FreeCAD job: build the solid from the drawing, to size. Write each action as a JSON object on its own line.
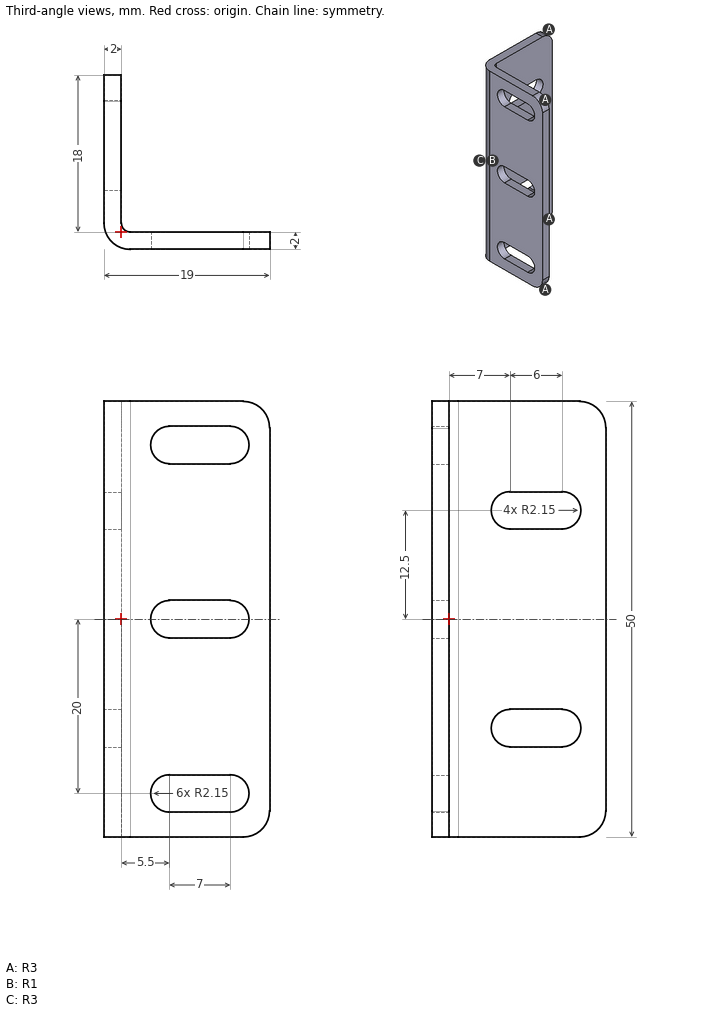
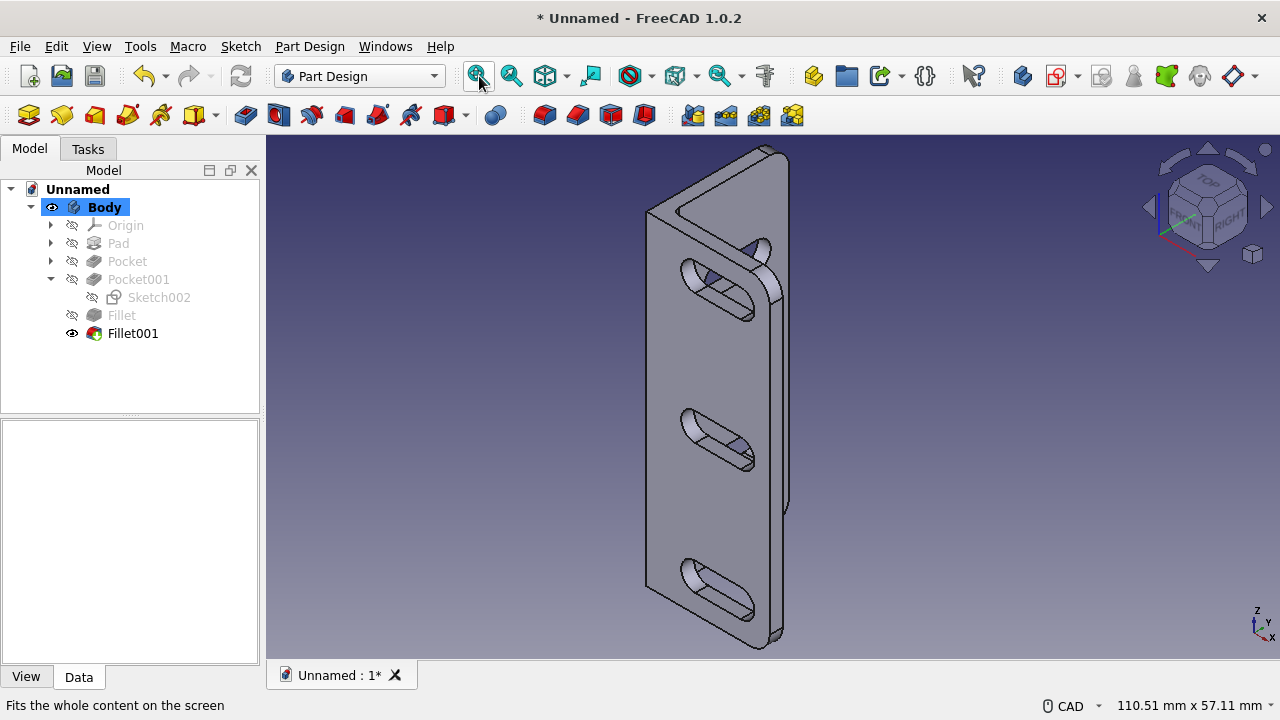
{"action": "key", "text": "1"}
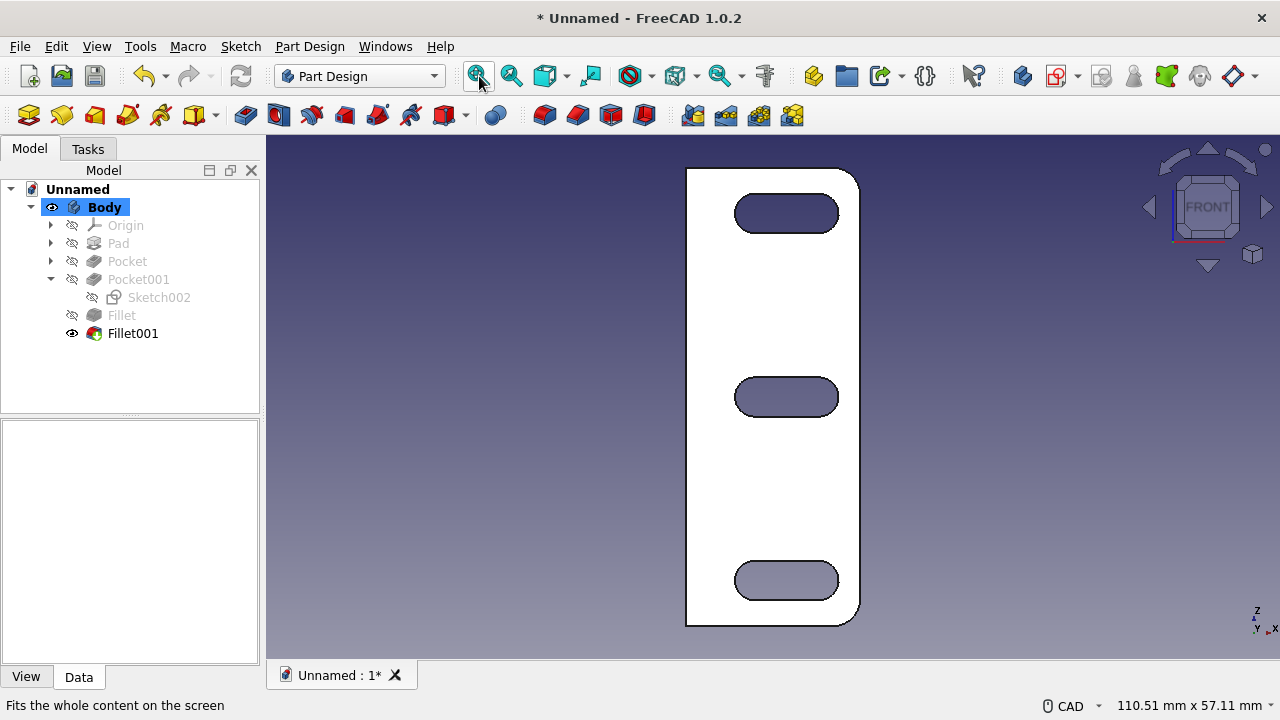
{"action": "left_click", "coordinate": [686, 396]}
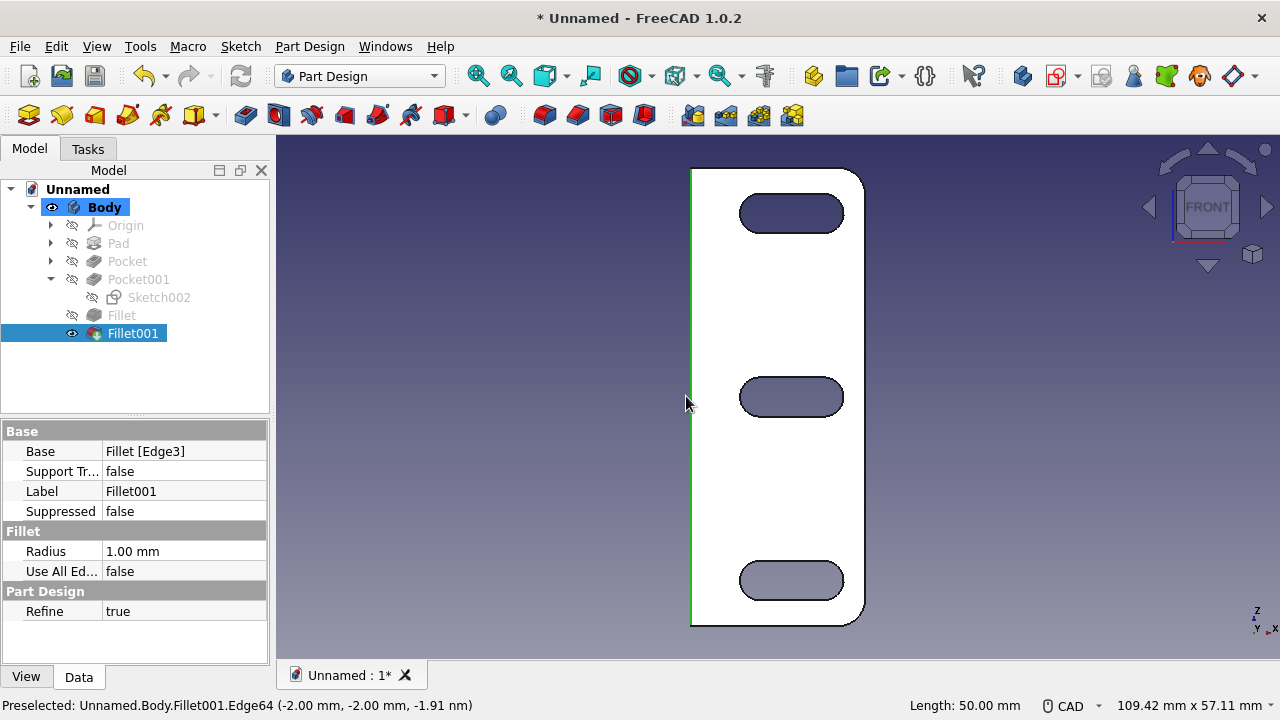
{"action": "left_click", "coordinate": [545, 116]}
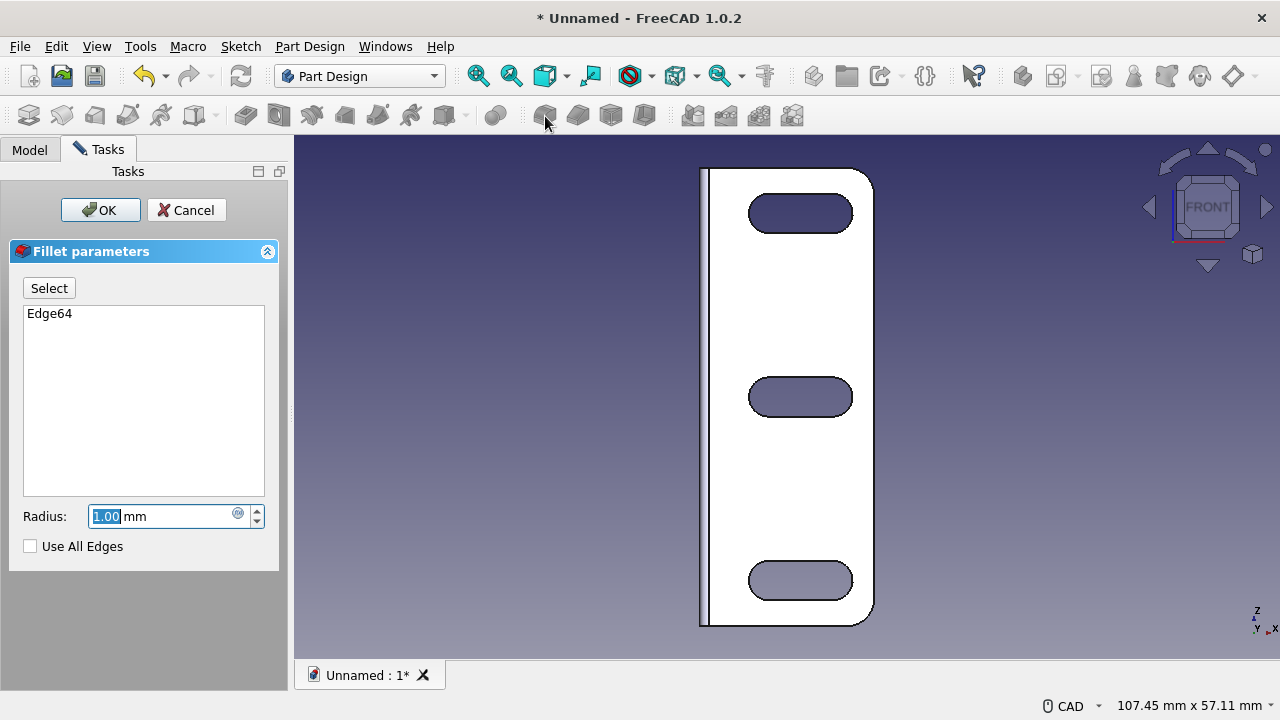
{"action": "type", "text": "3"}
{"action": "key", "text": "Tab"}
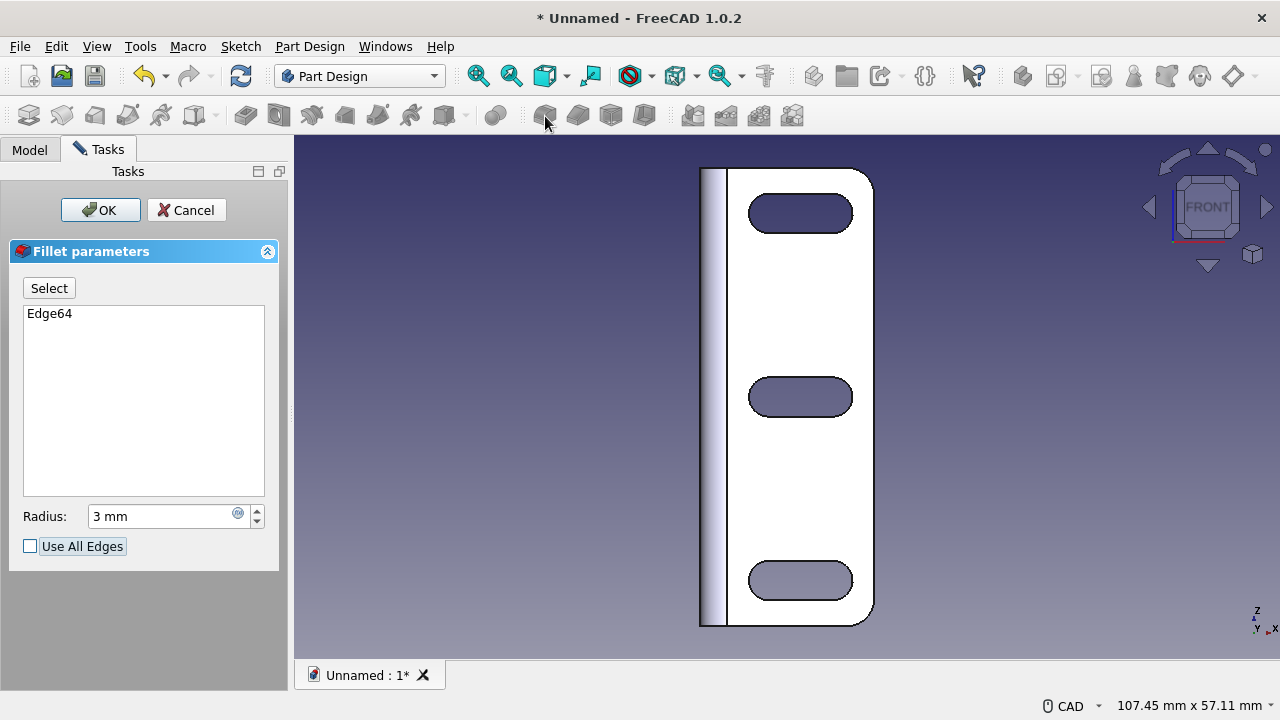
{"action": "left_click", "coordinate": [101, 210]}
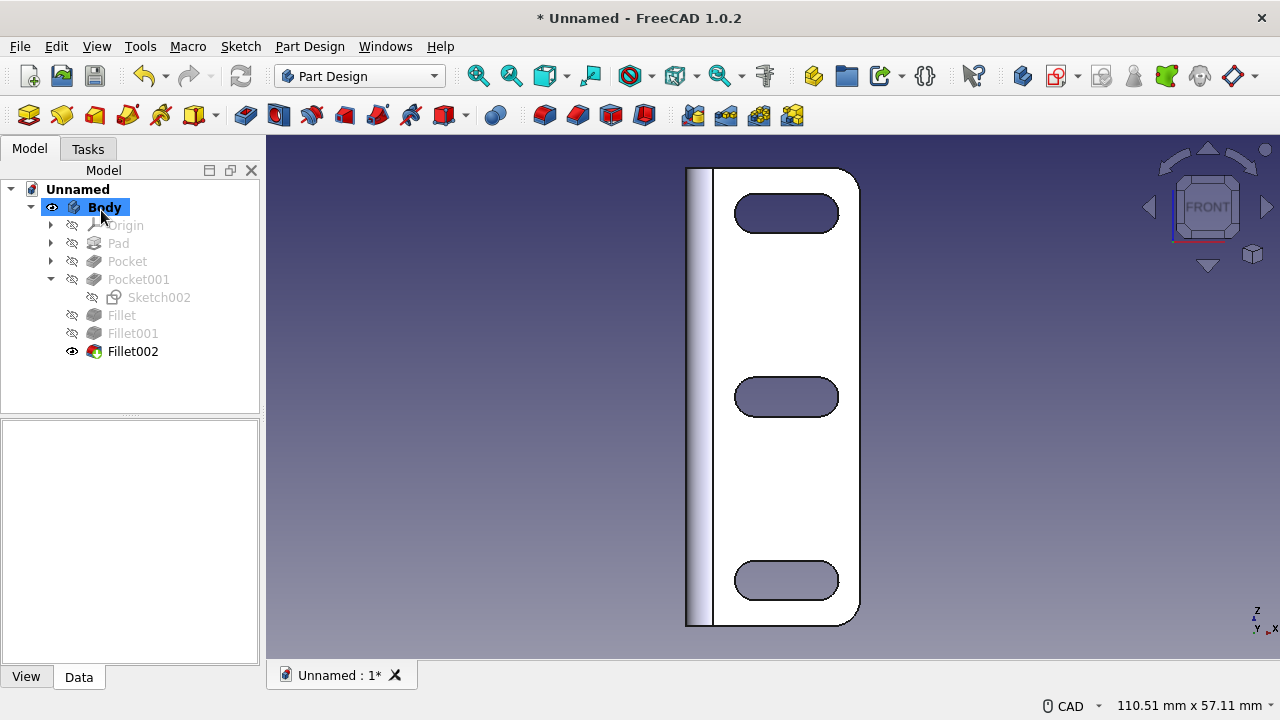
{"action": "key", "text": "0"}